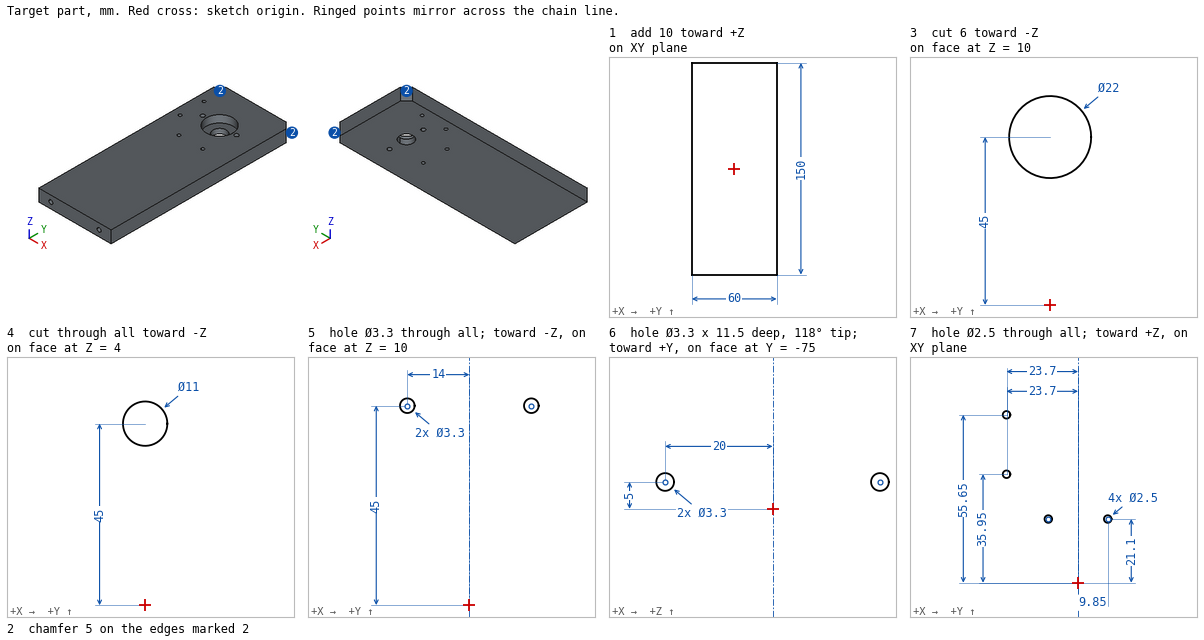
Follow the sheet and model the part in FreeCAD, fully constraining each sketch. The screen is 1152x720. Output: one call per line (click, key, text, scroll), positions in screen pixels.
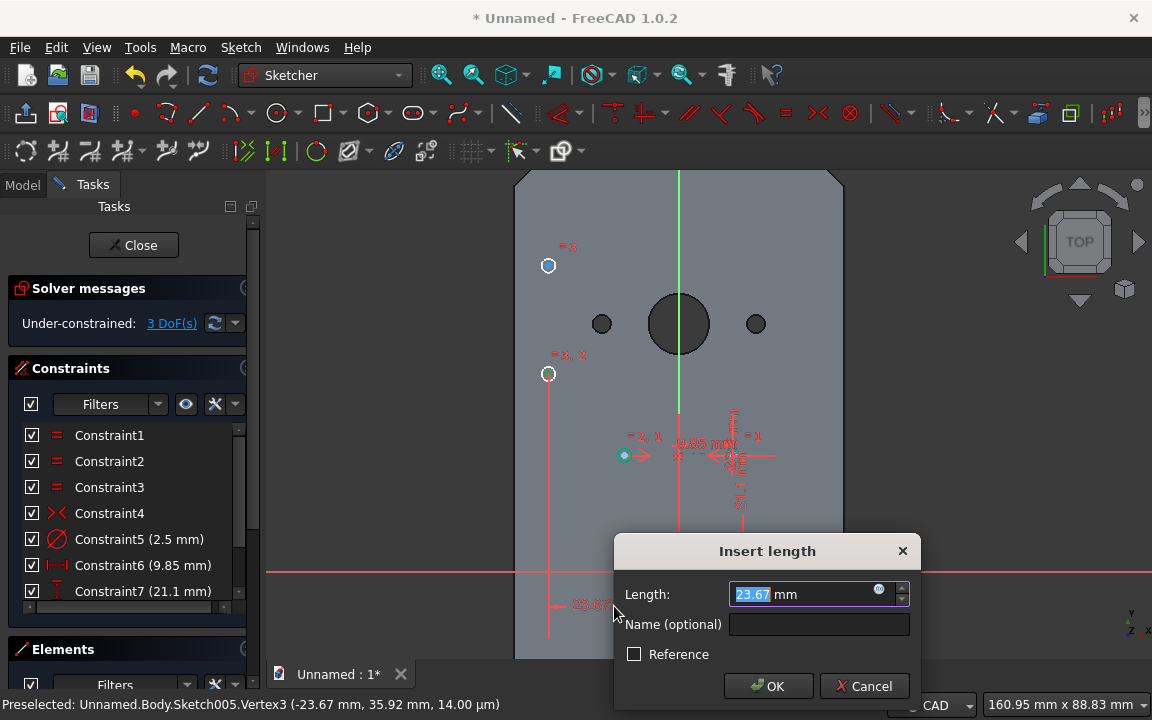
text(23.7)
key(Return)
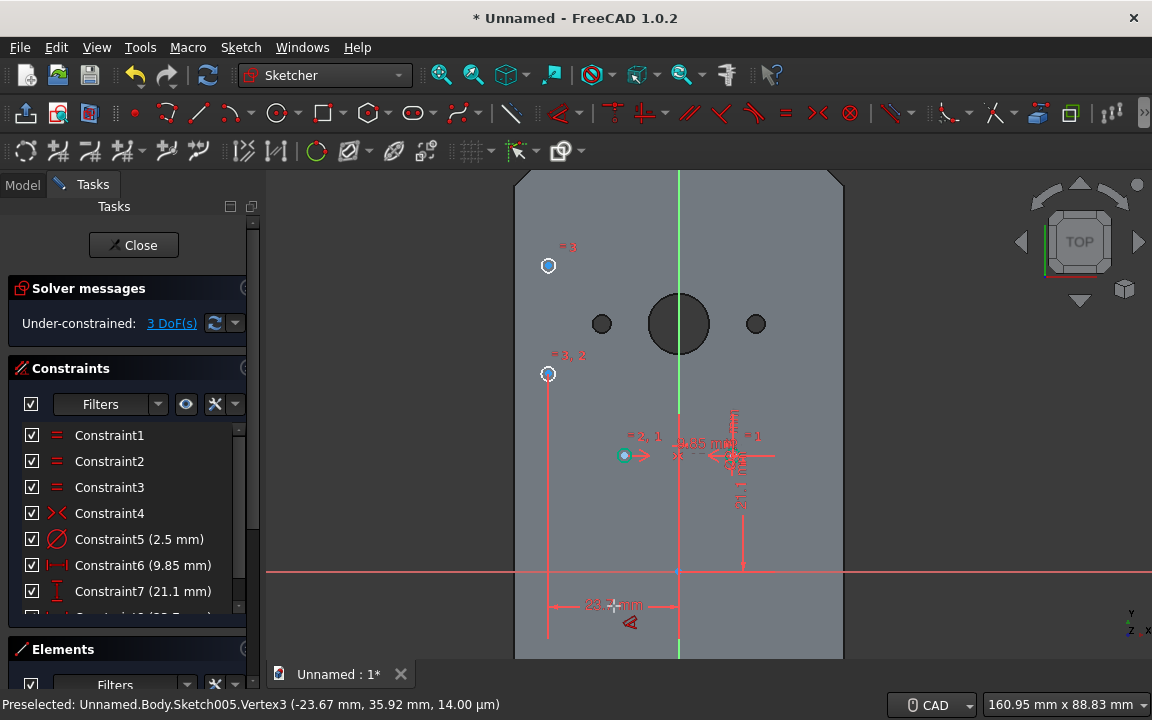
click(549, 266)
click(614, 232)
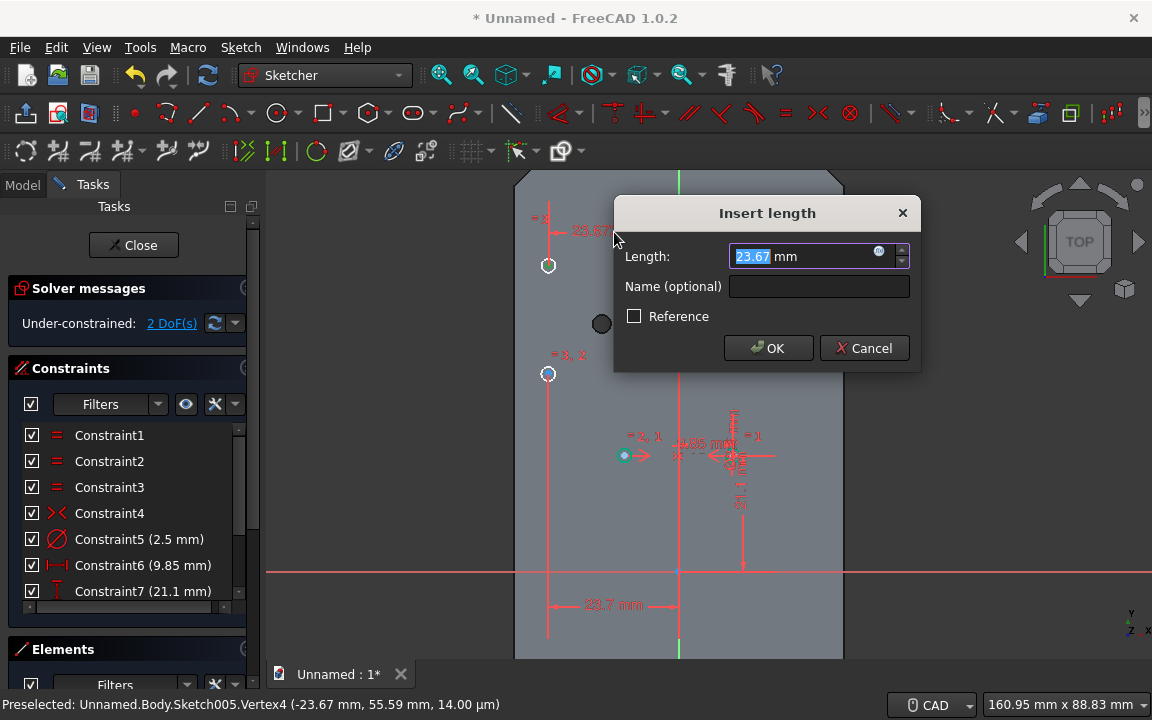
text(23.7)
key(Return)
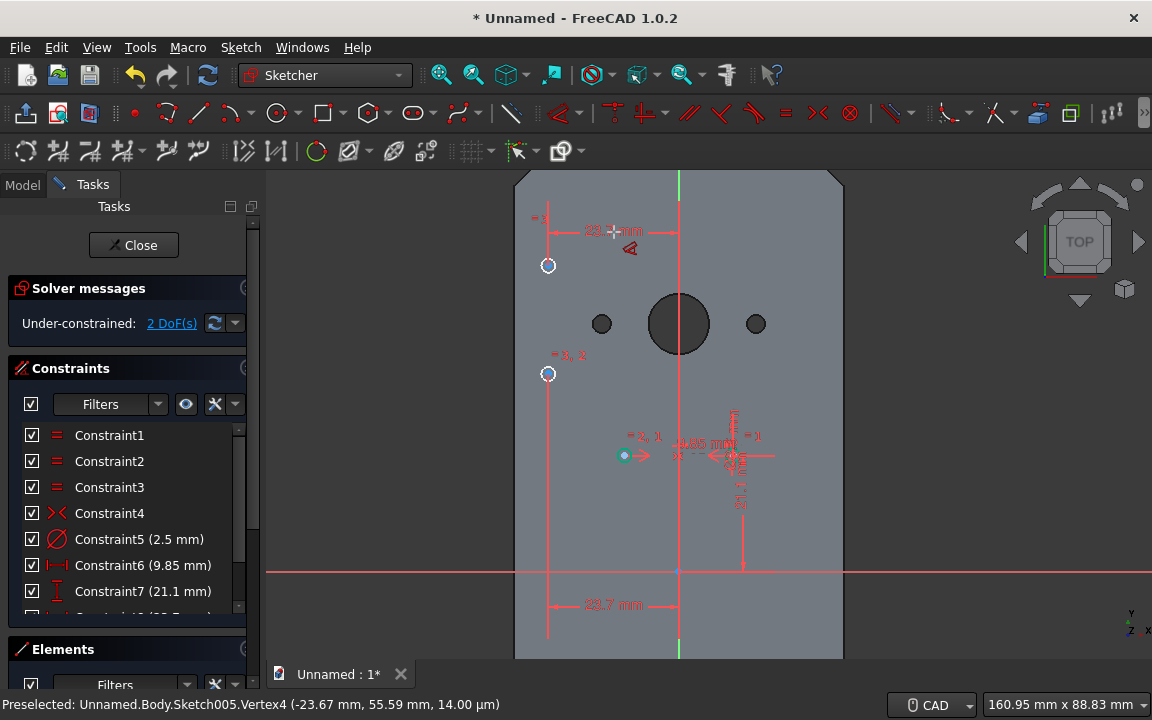
click(548, 374)
click(514, 473)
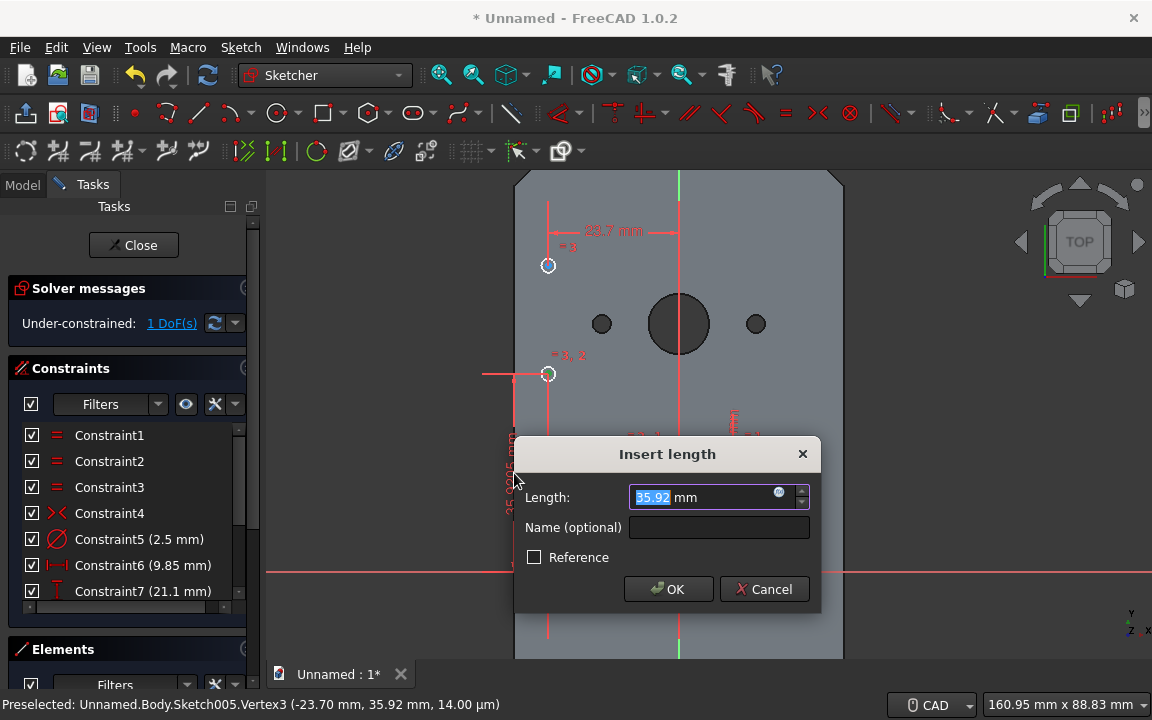
text(35.95)
key(Return)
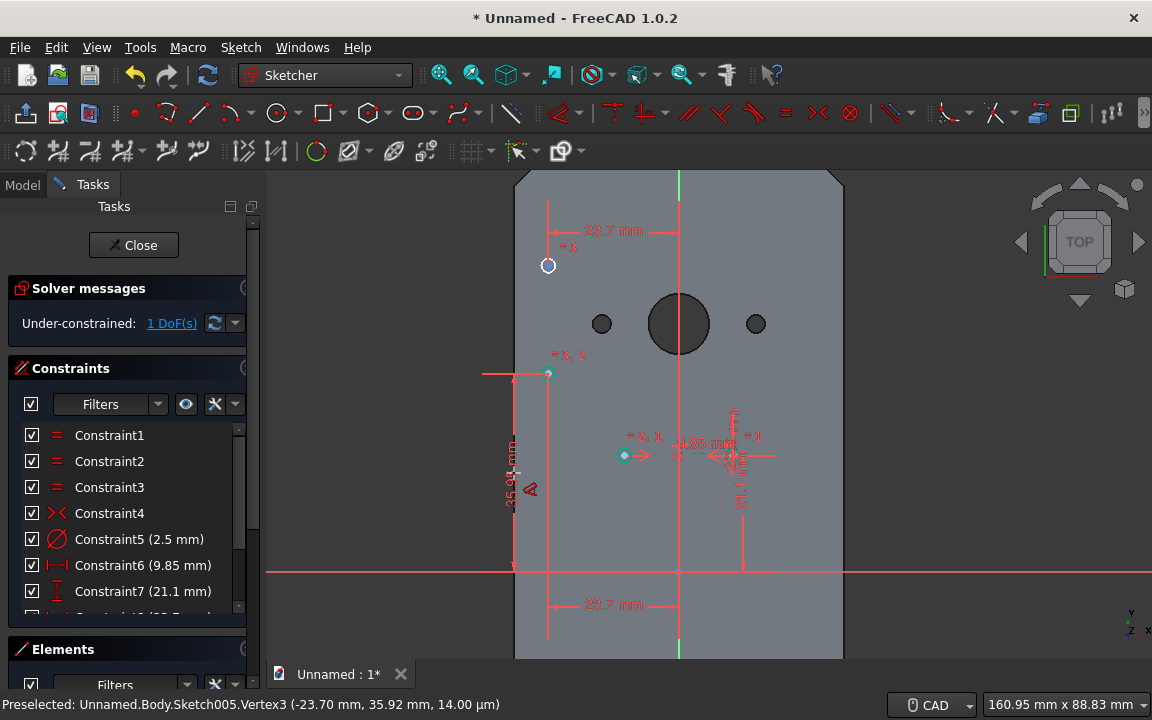
click(548, 266)
click(514, 419)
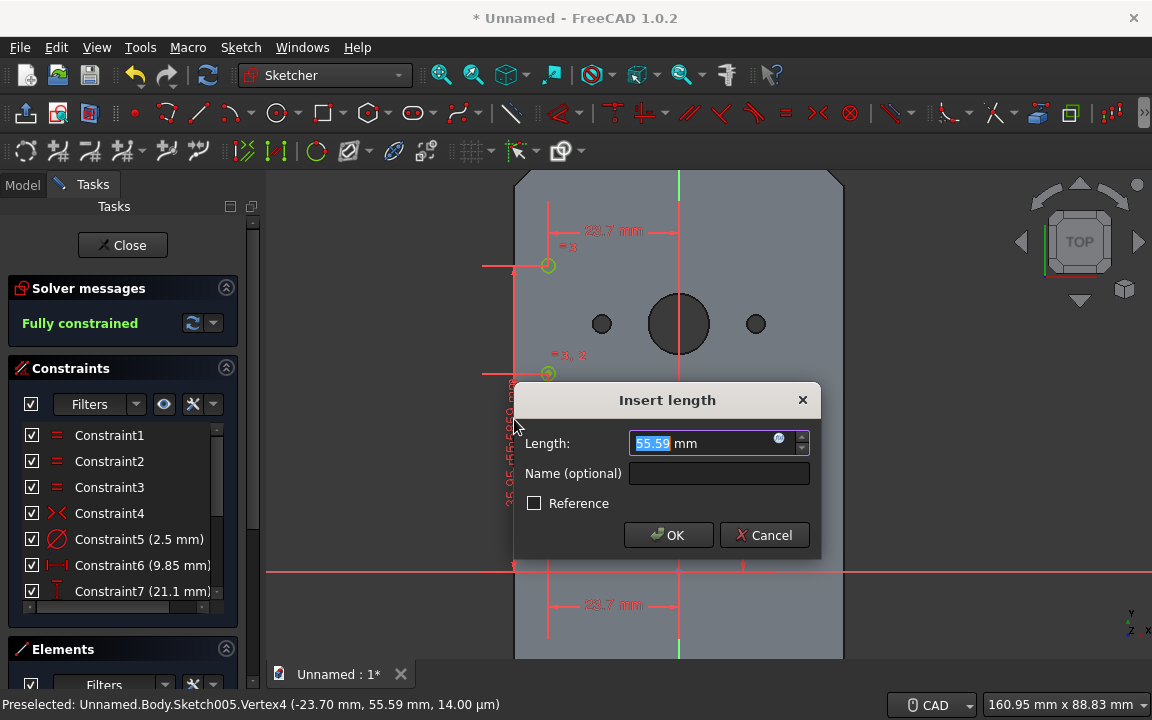
text(55.65)
key(Return)
key(Escape)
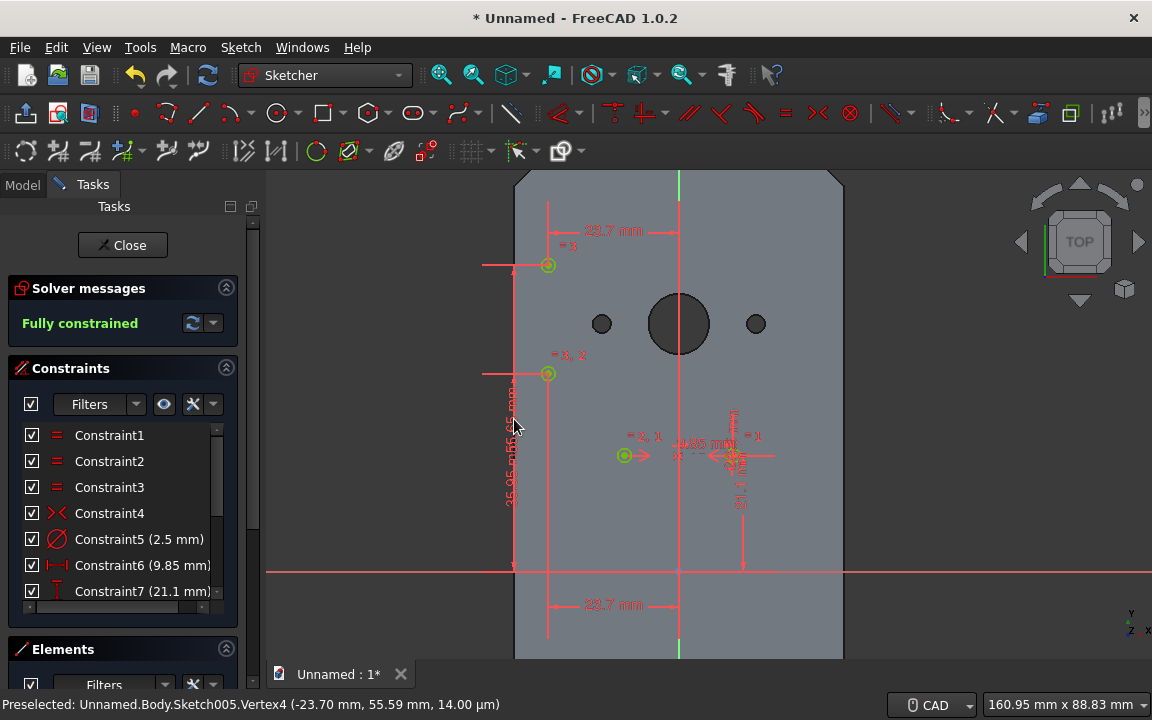
click(123, 245)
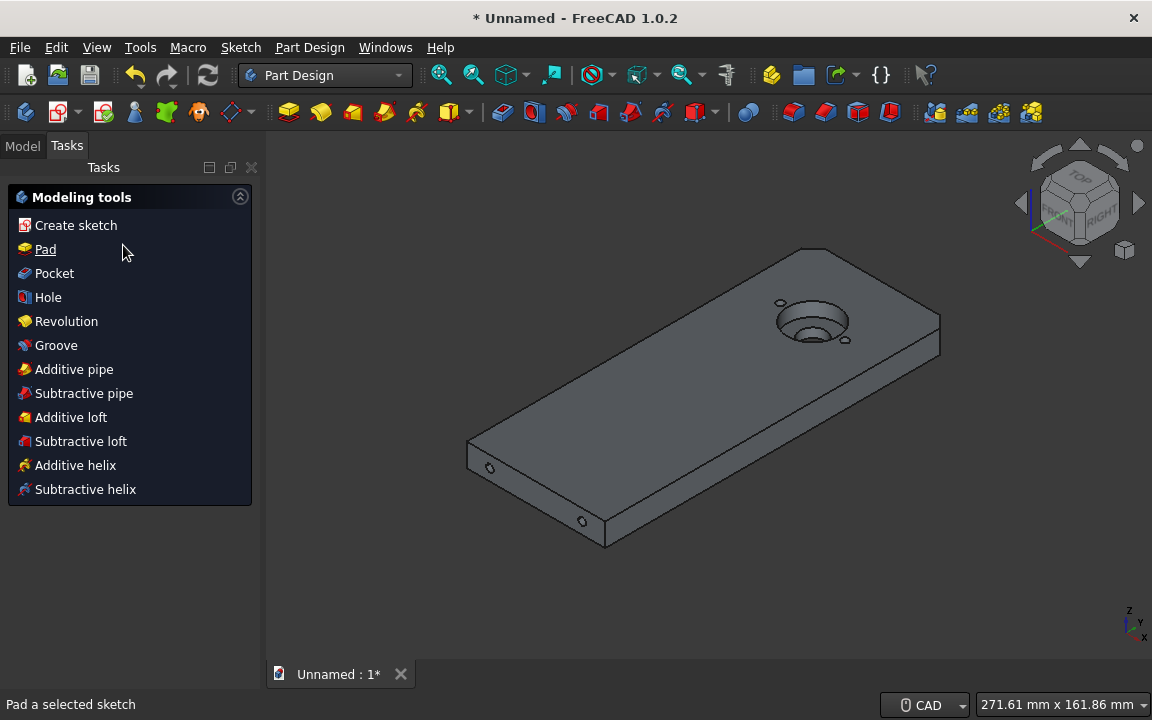
click(536, 112)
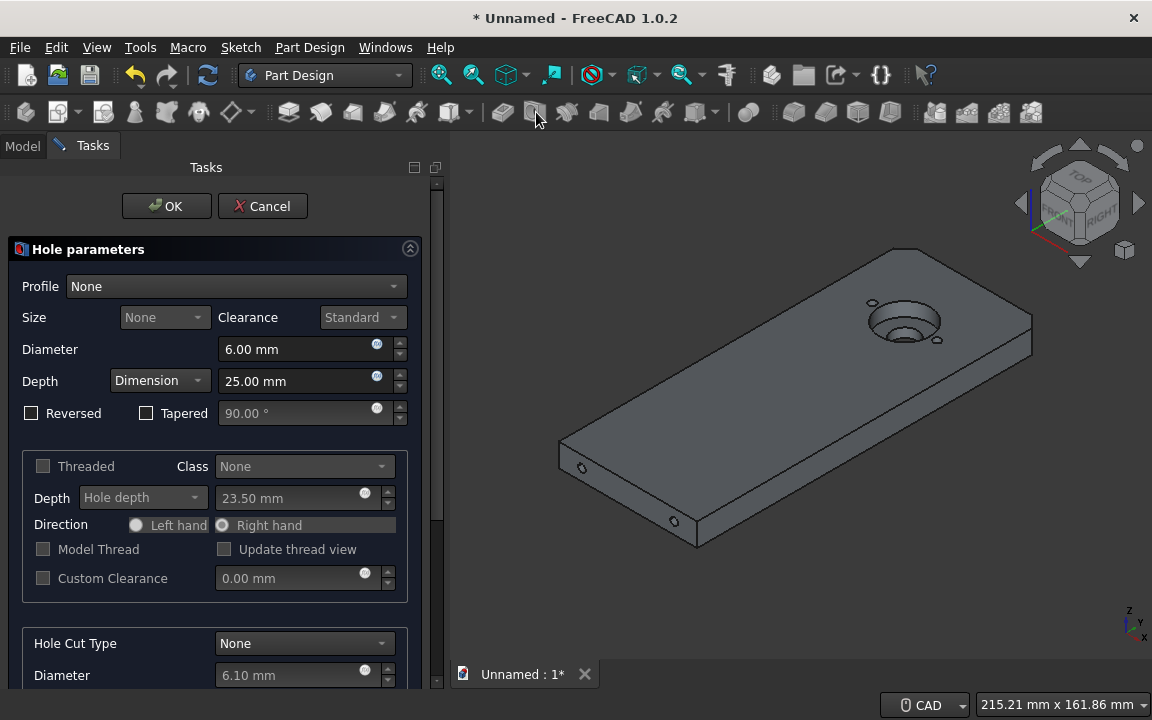
triple_click(305, 349)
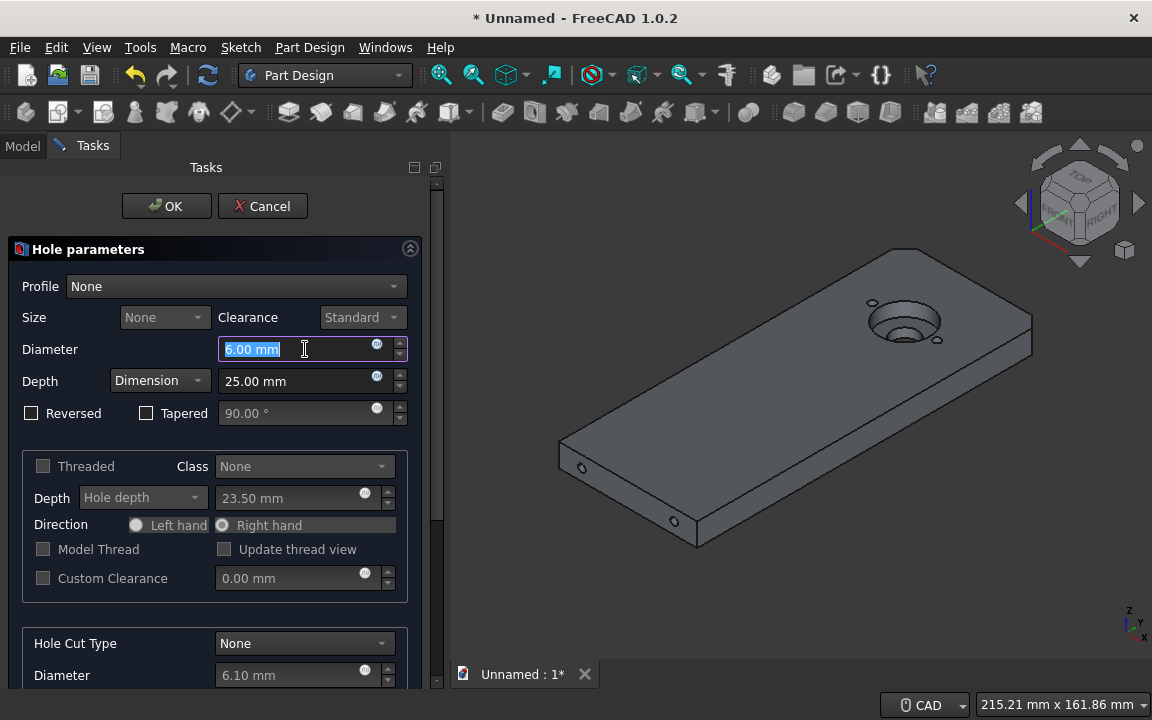
text(2.5)
key(Tab)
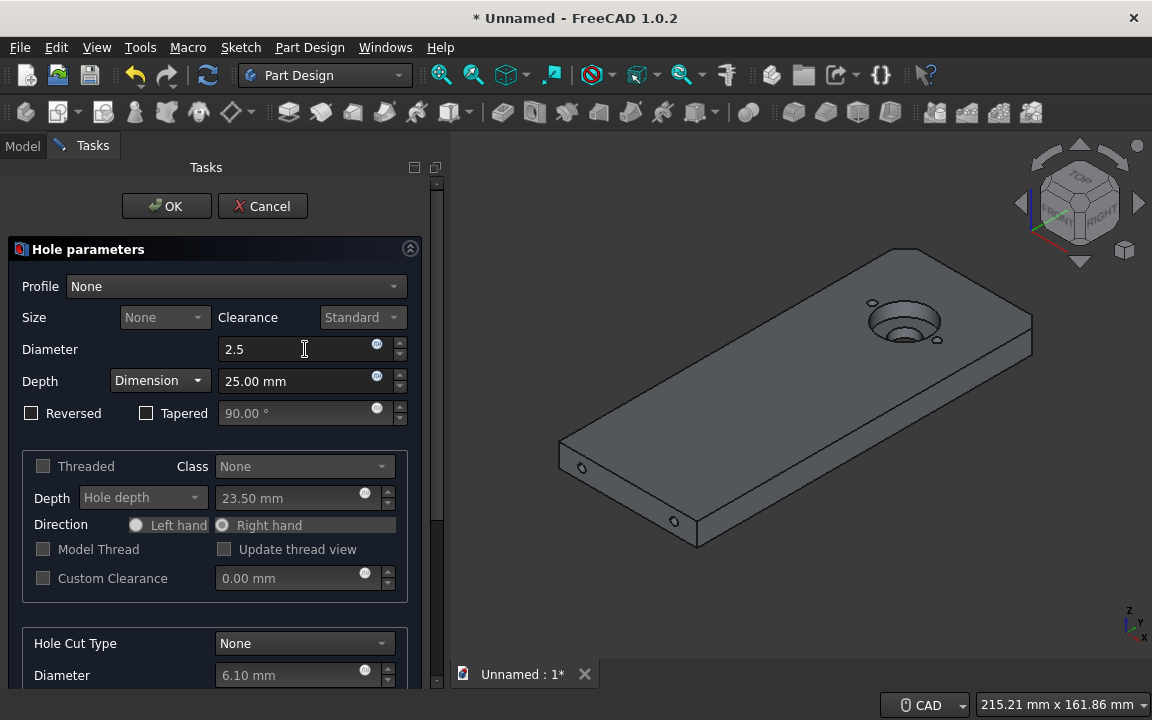
click(161, 380)